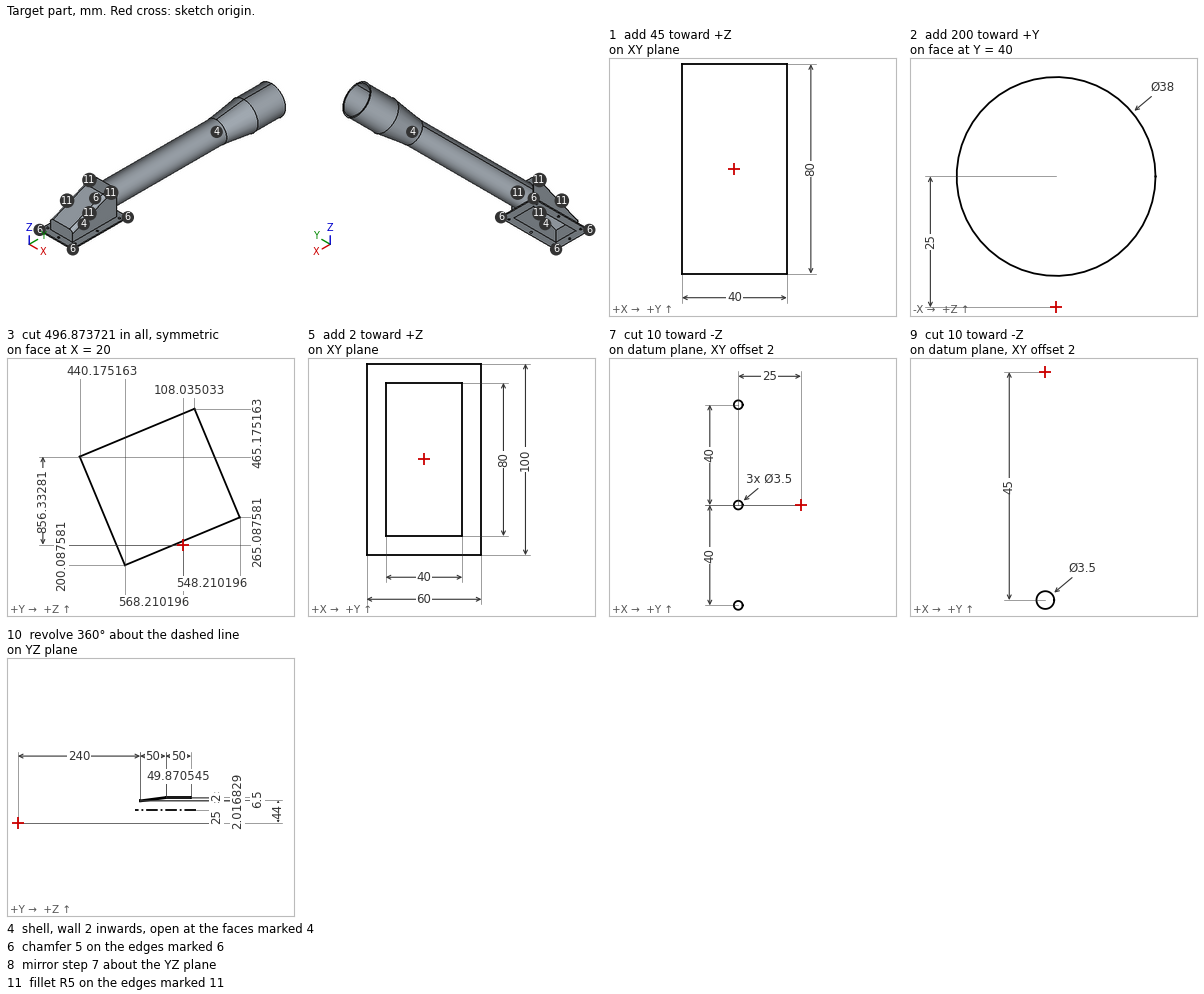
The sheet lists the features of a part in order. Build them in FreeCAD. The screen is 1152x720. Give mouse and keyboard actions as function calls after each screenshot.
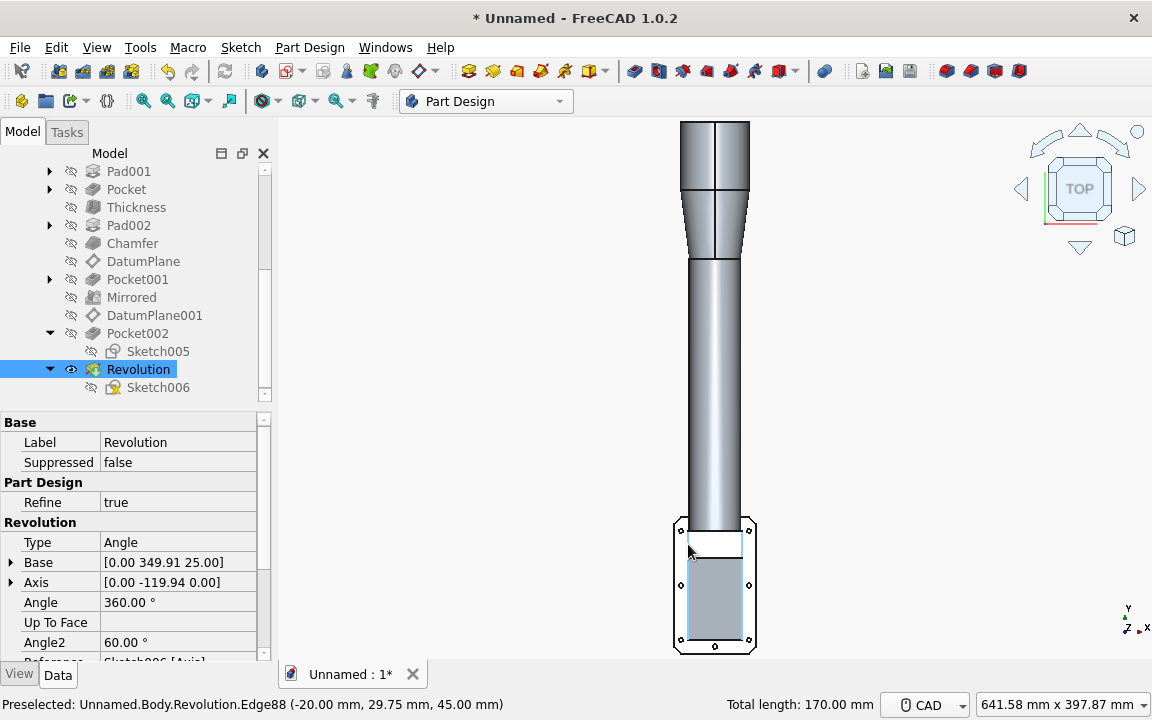
click(948, 72)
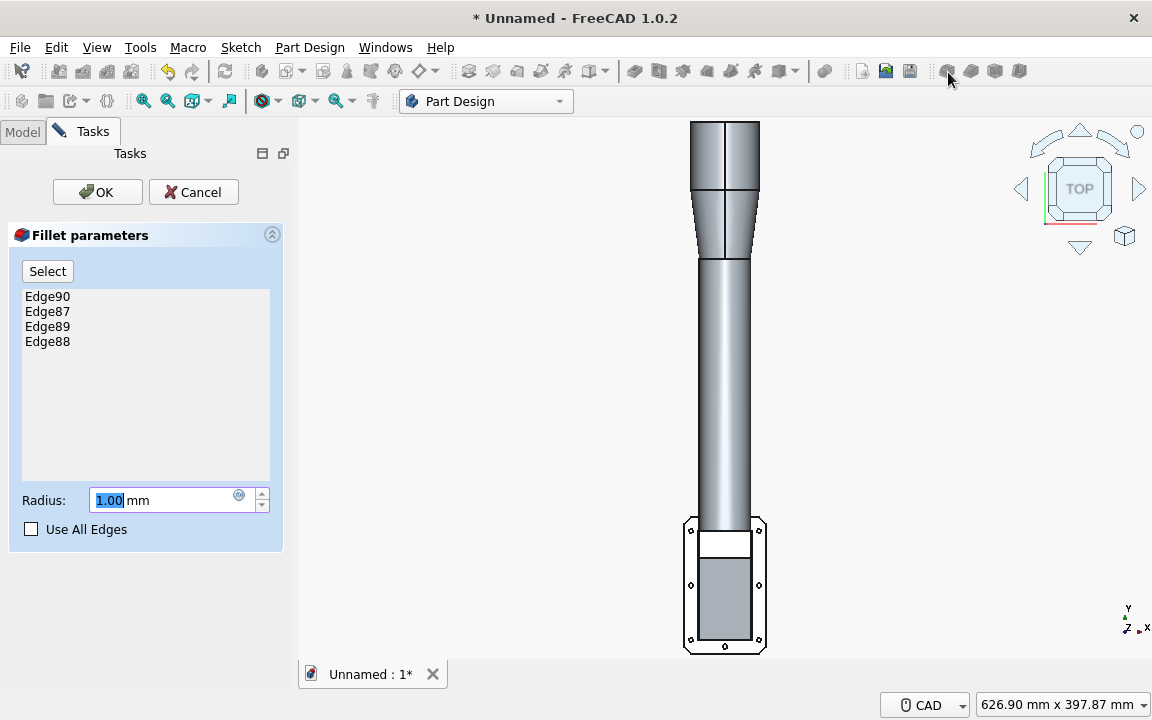
text(5)
key(Tab)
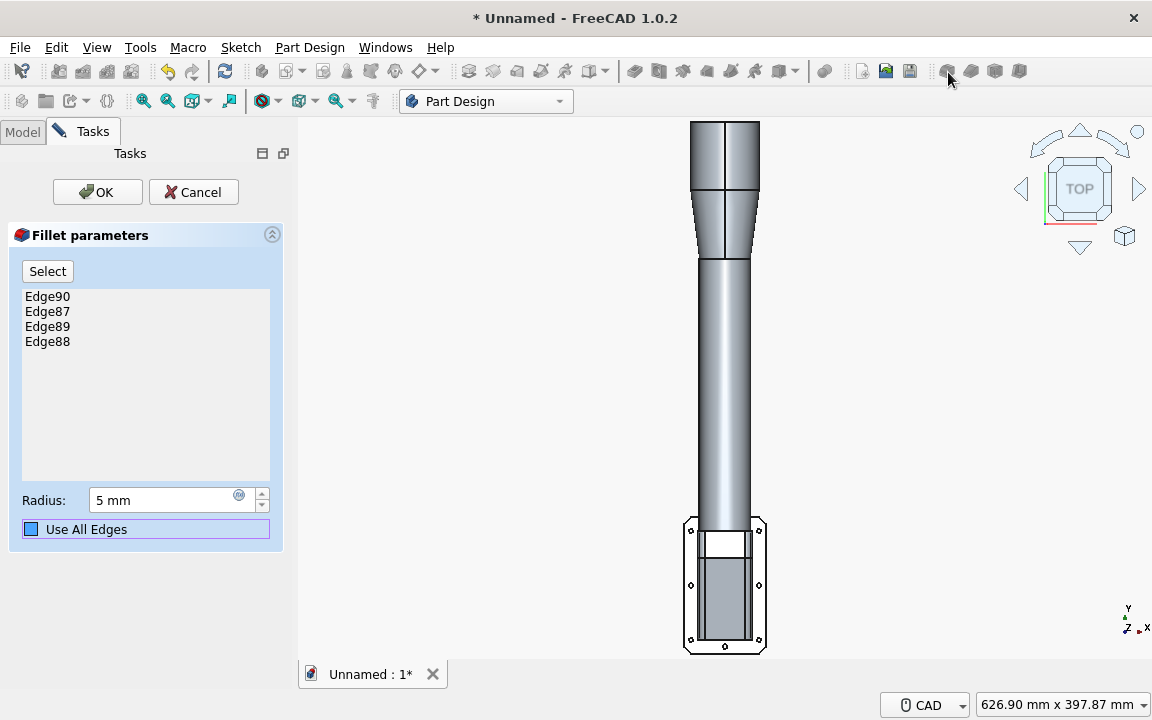
click(98, 192)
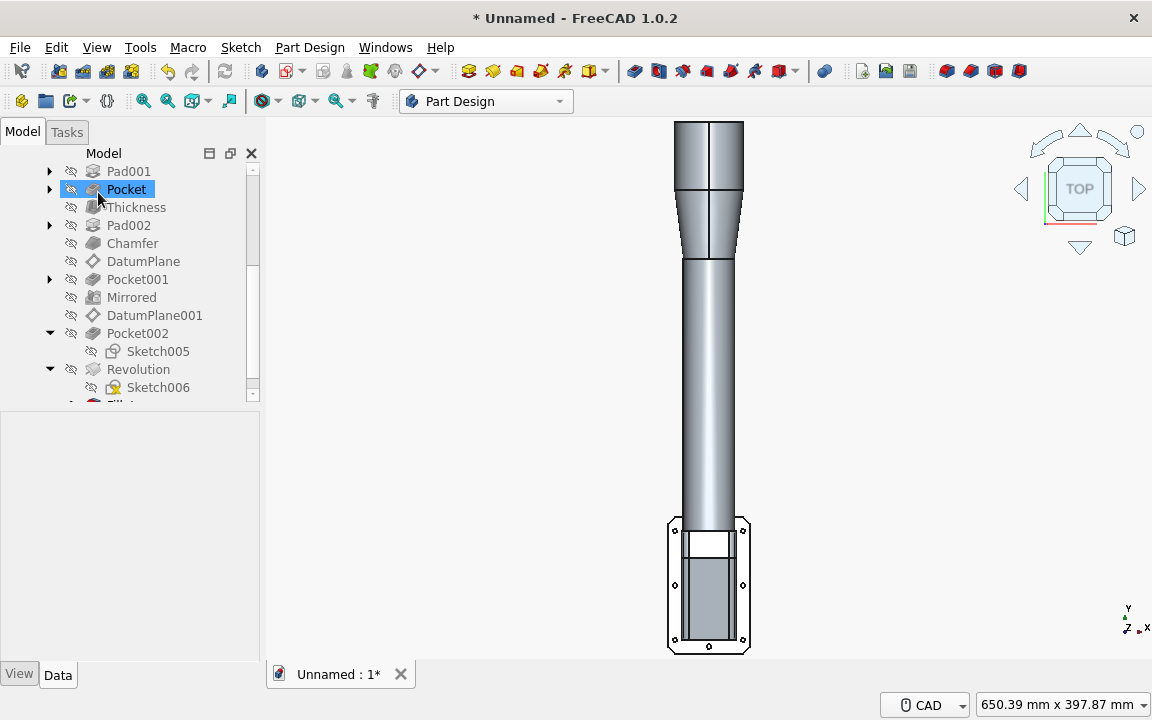
key(0)